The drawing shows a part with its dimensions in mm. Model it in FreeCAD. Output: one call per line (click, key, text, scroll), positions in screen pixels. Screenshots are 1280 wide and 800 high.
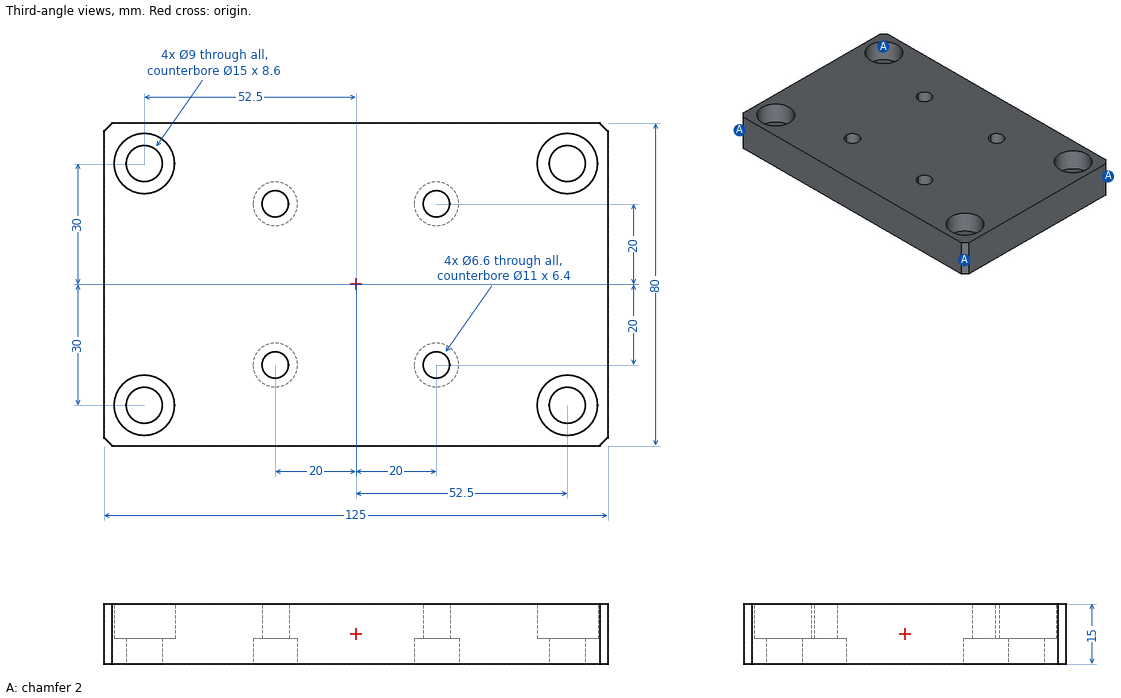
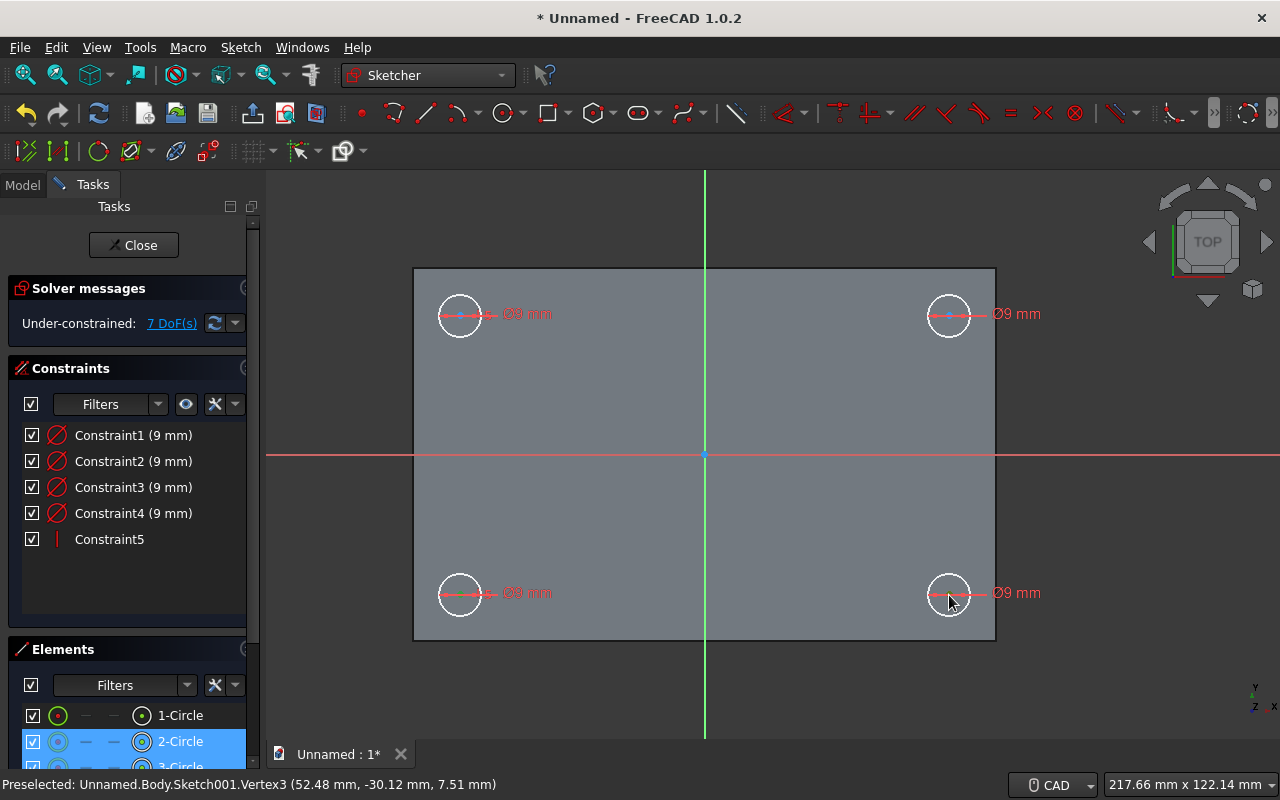
click(892, 114)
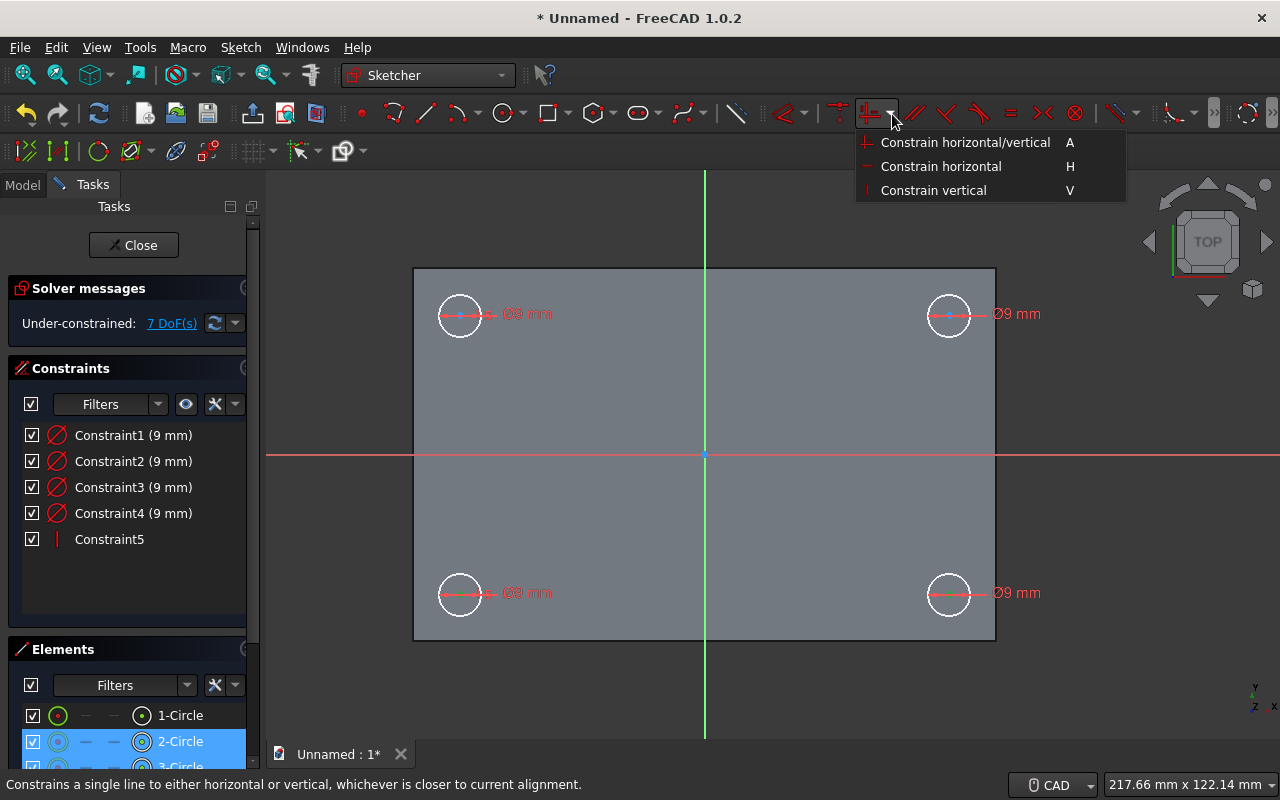
click(991, 166)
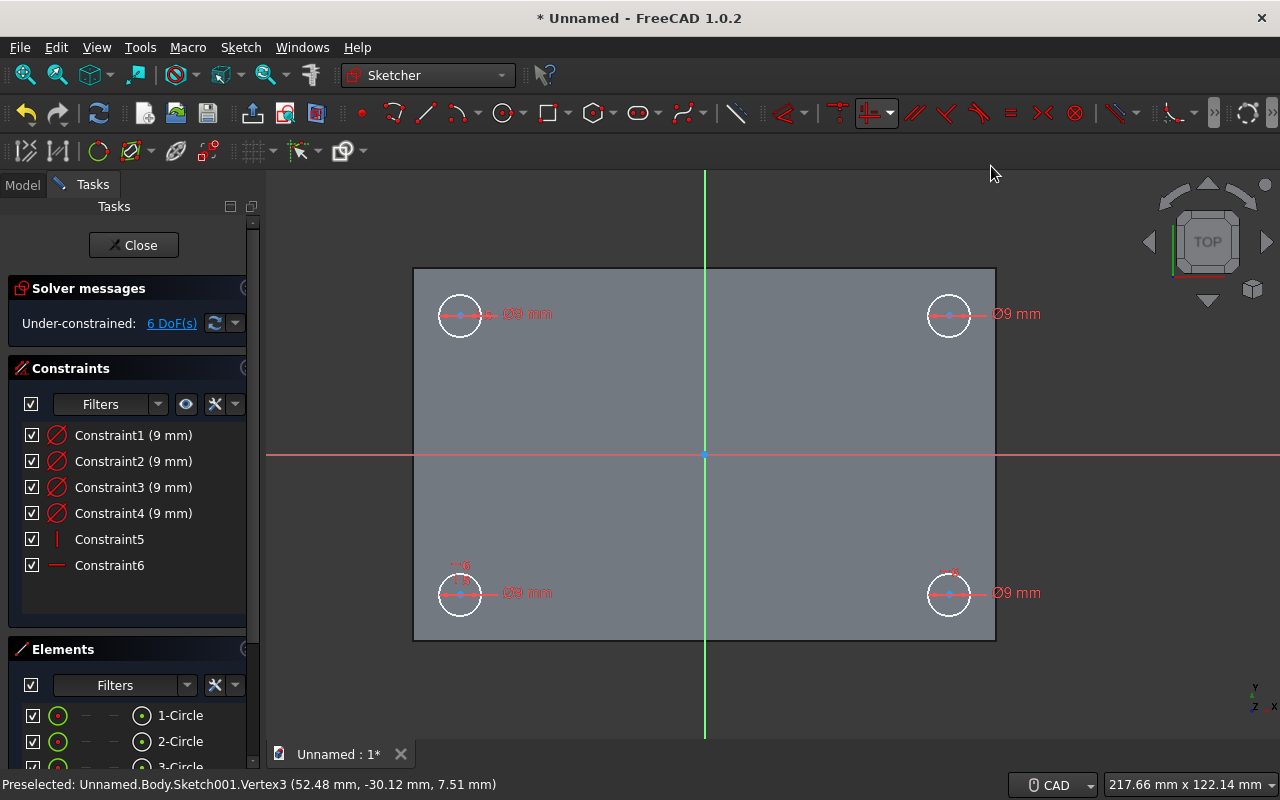
click(949, 595)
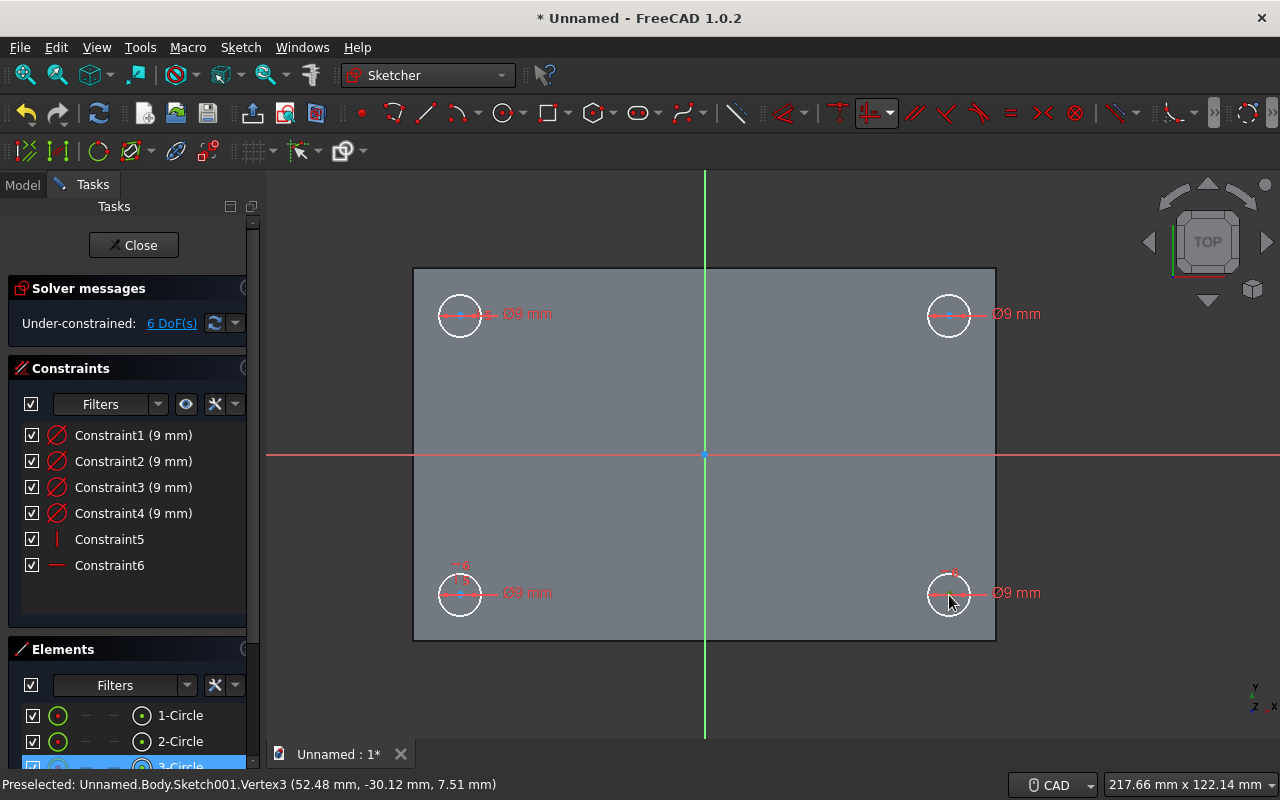
click(949, 316)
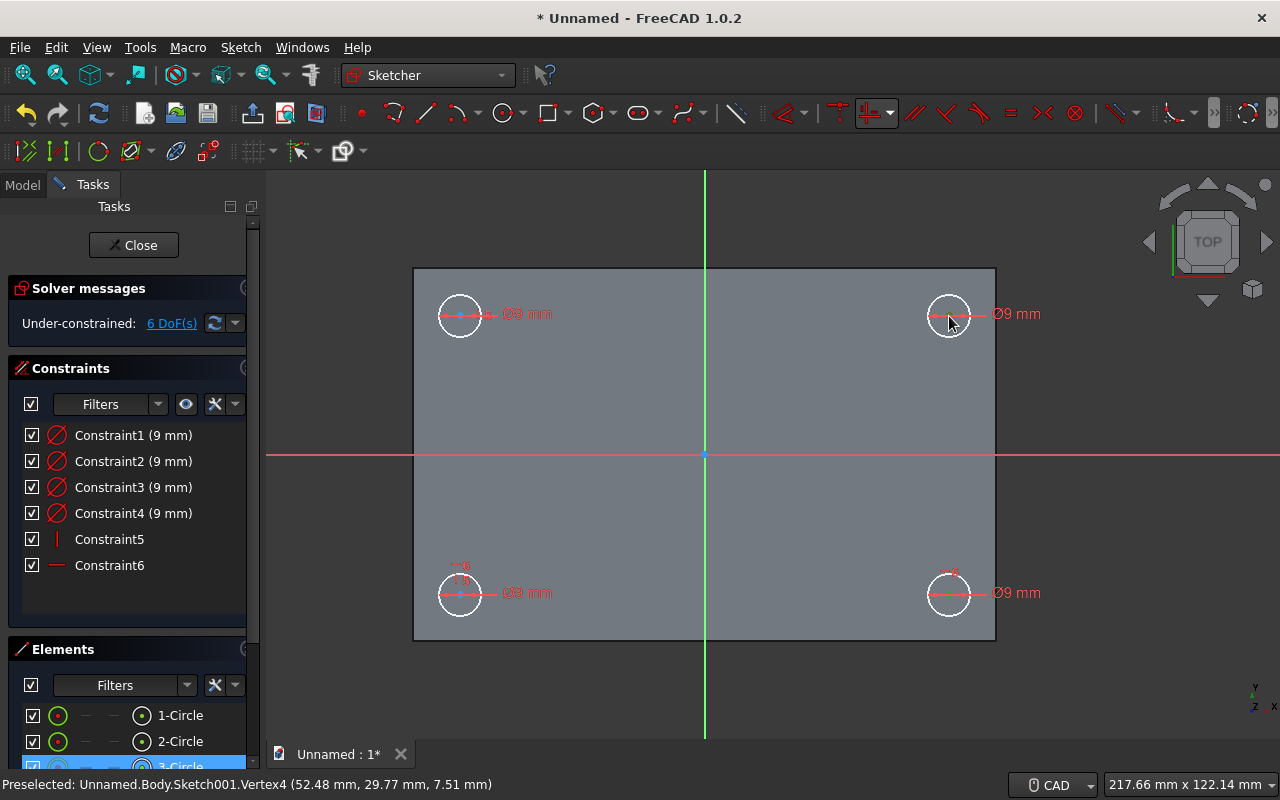
key(v)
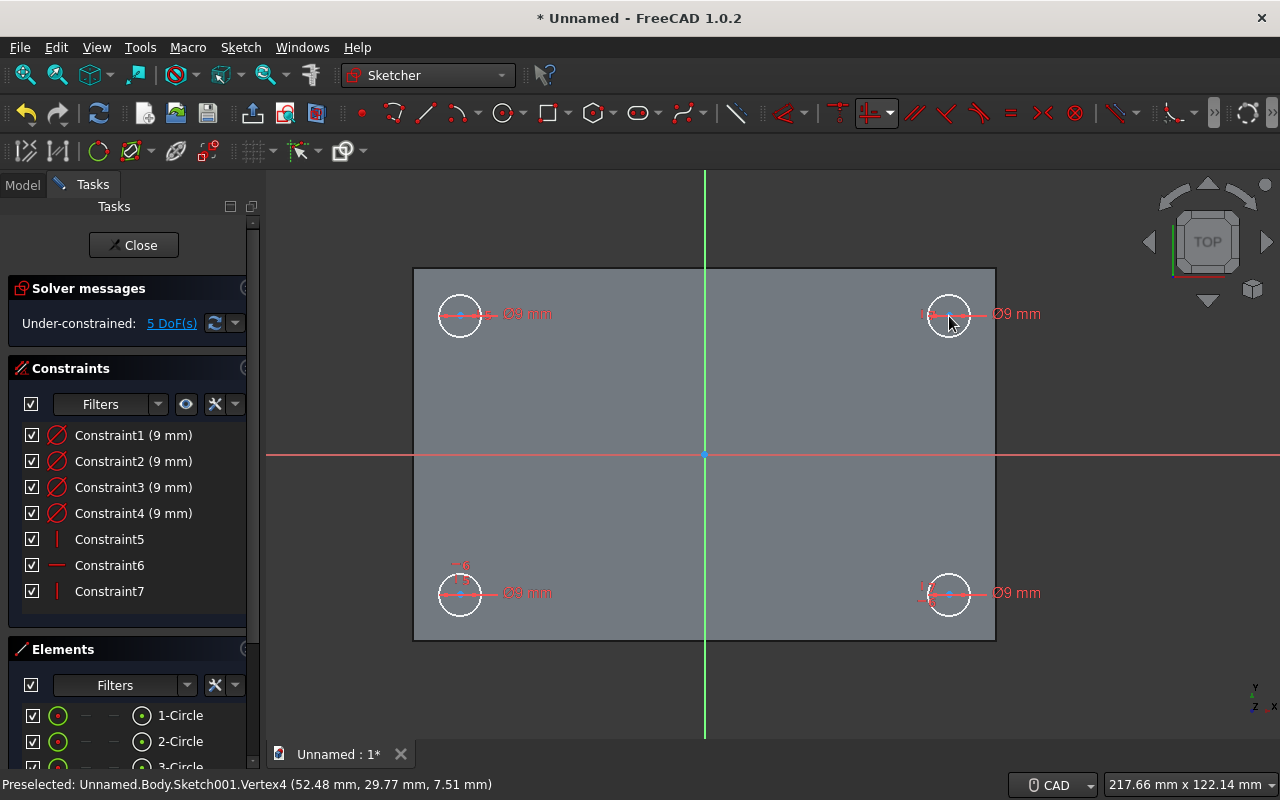
click(460, 316)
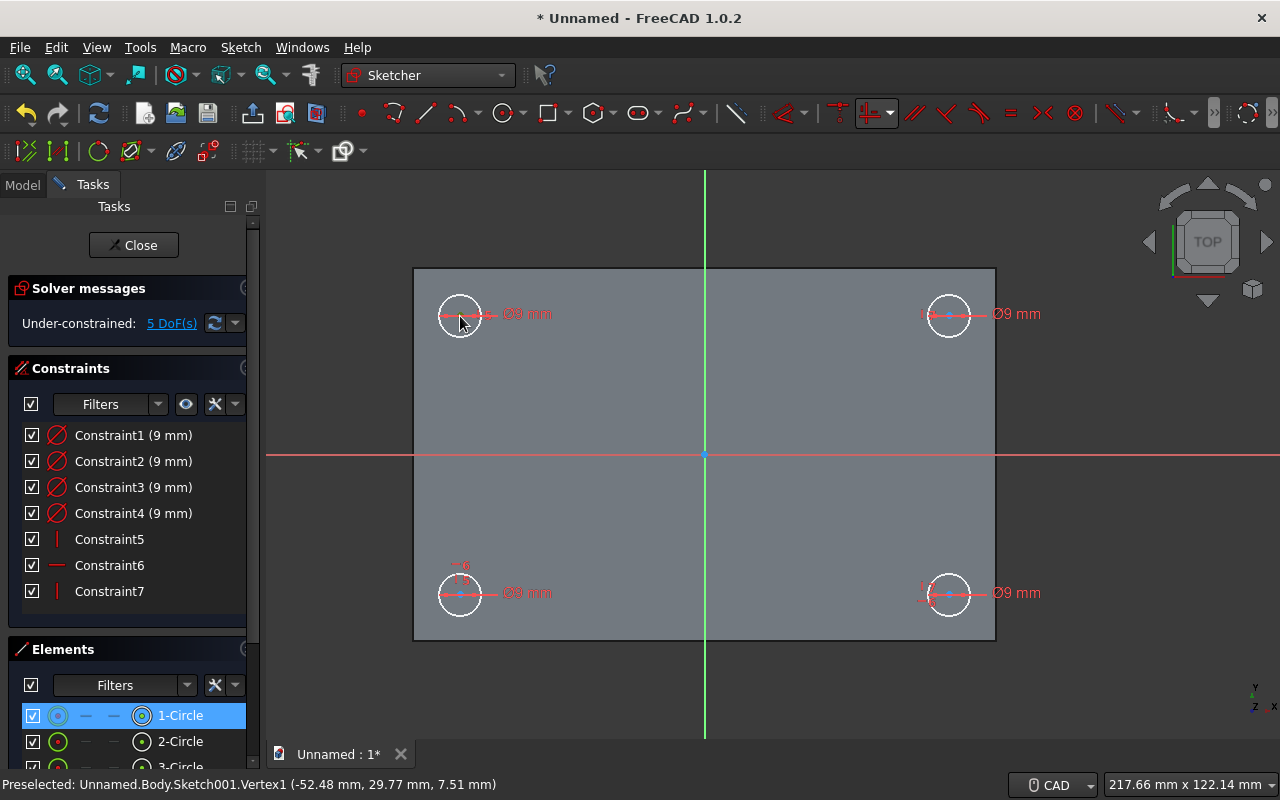
click(949, 316)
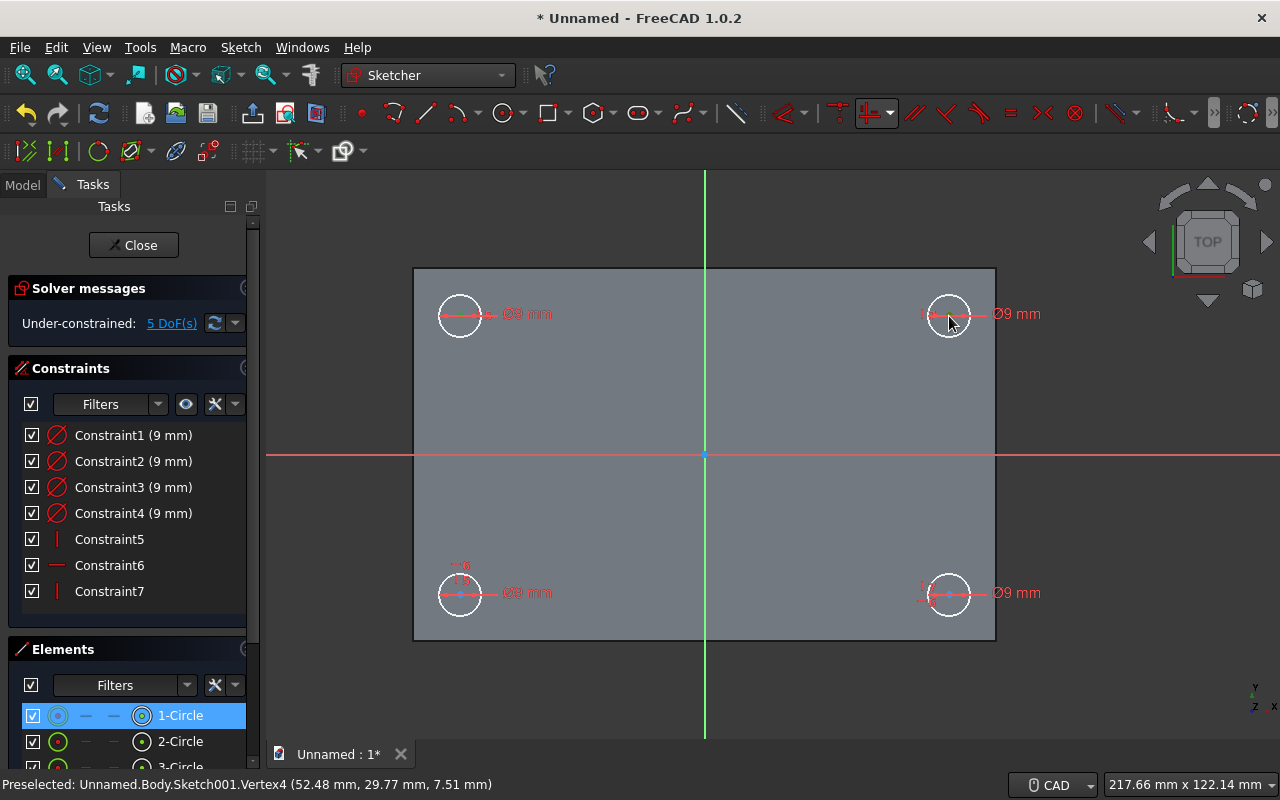
key(h)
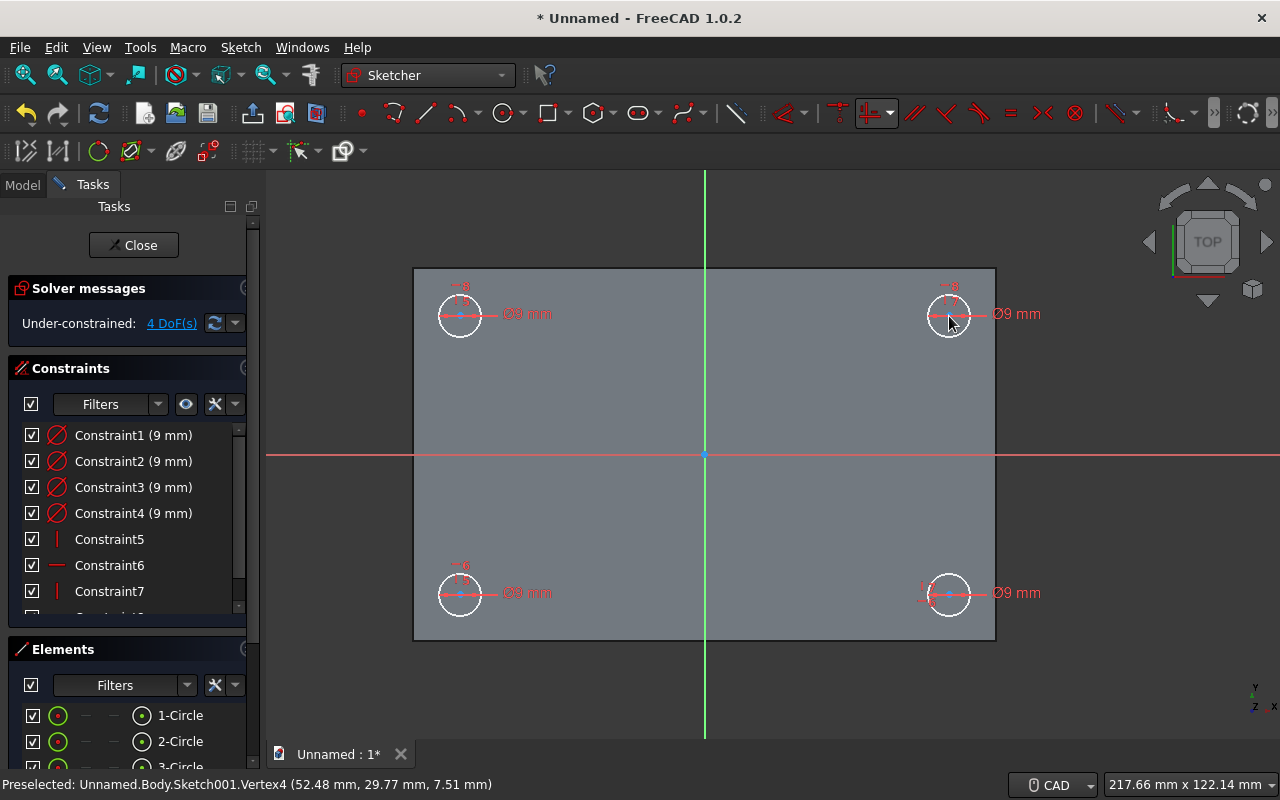
click(784, 114)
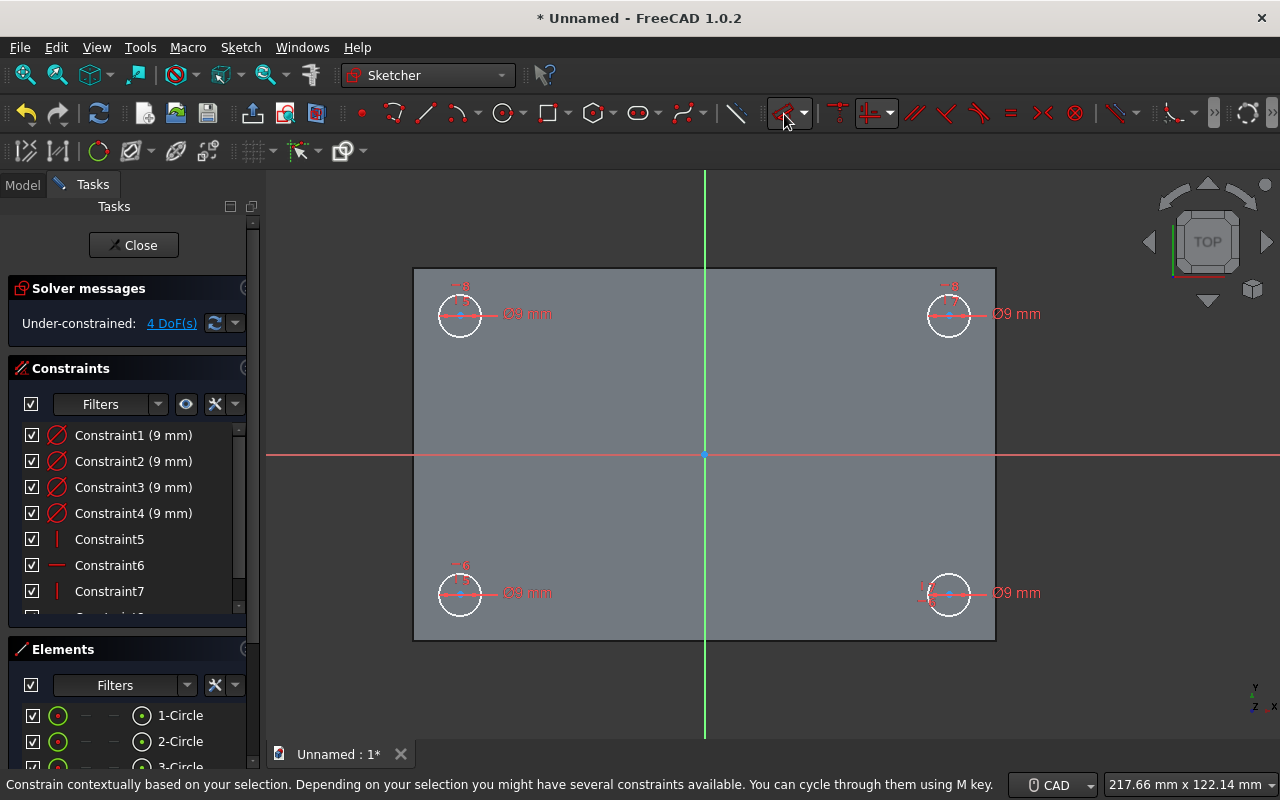
click(460, 316)
click(426, 385)